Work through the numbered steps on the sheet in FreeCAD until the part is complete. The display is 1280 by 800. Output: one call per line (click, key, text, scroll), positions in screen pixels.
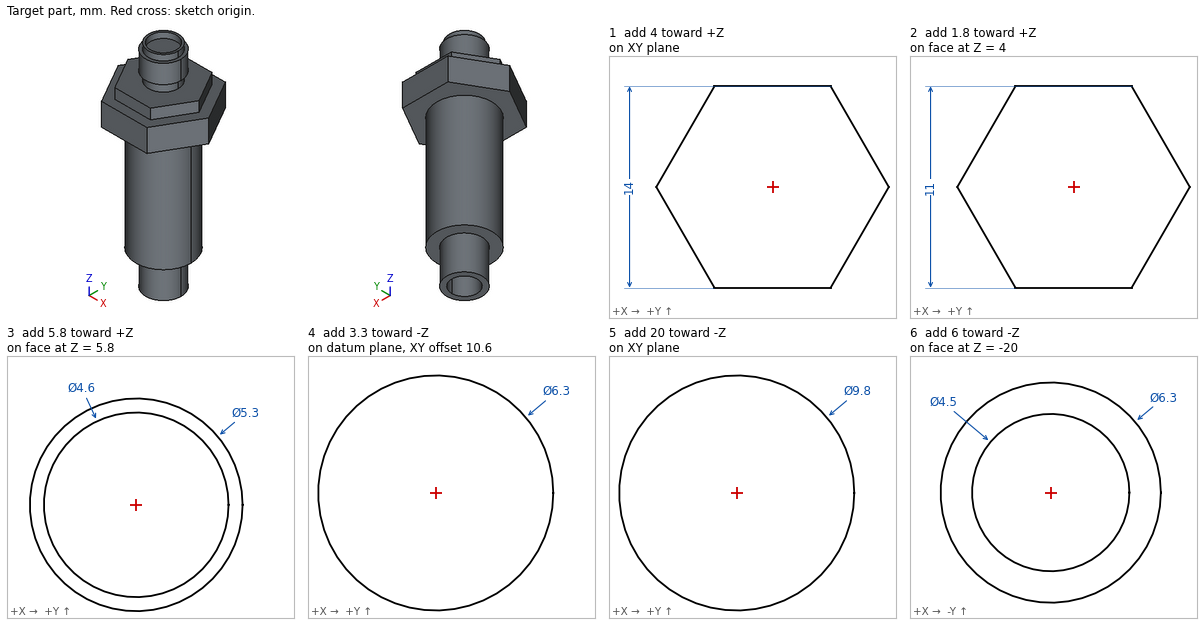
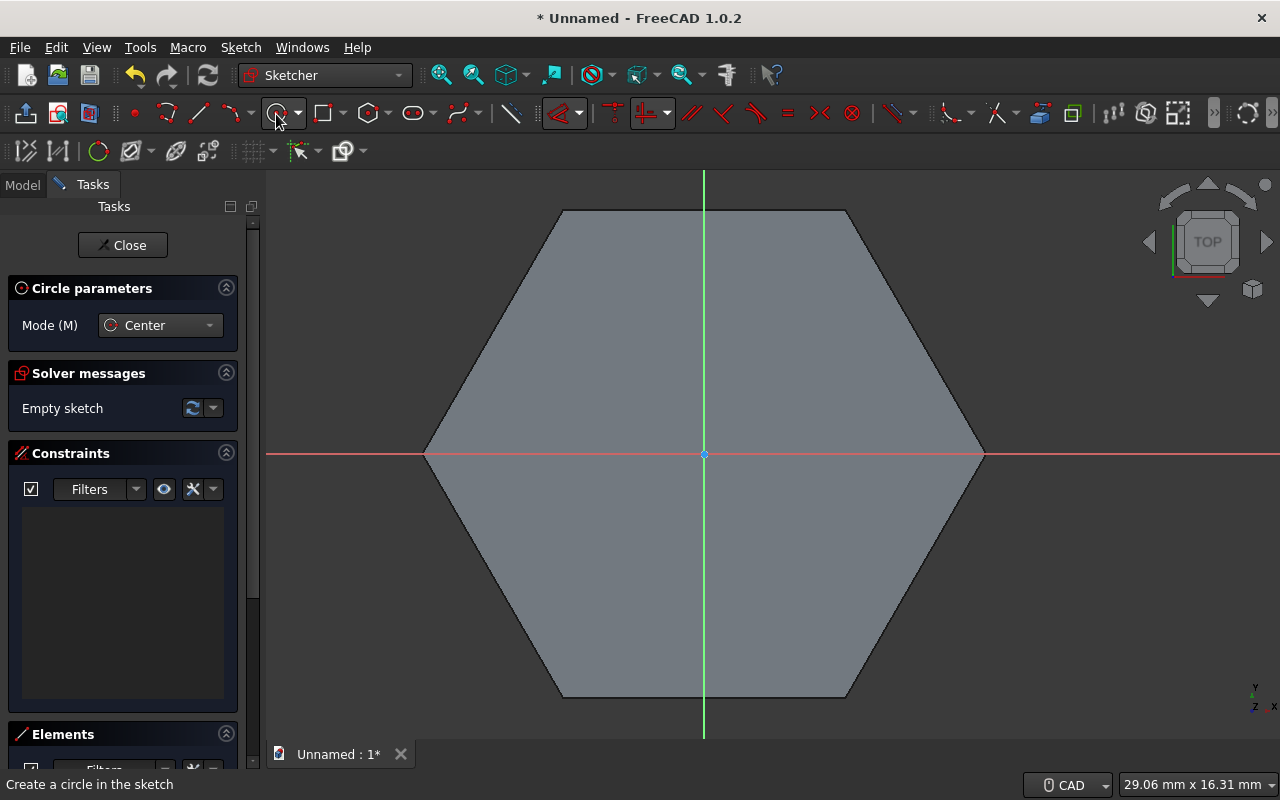
click(704, 454)
click(825, 333)
key(Escape)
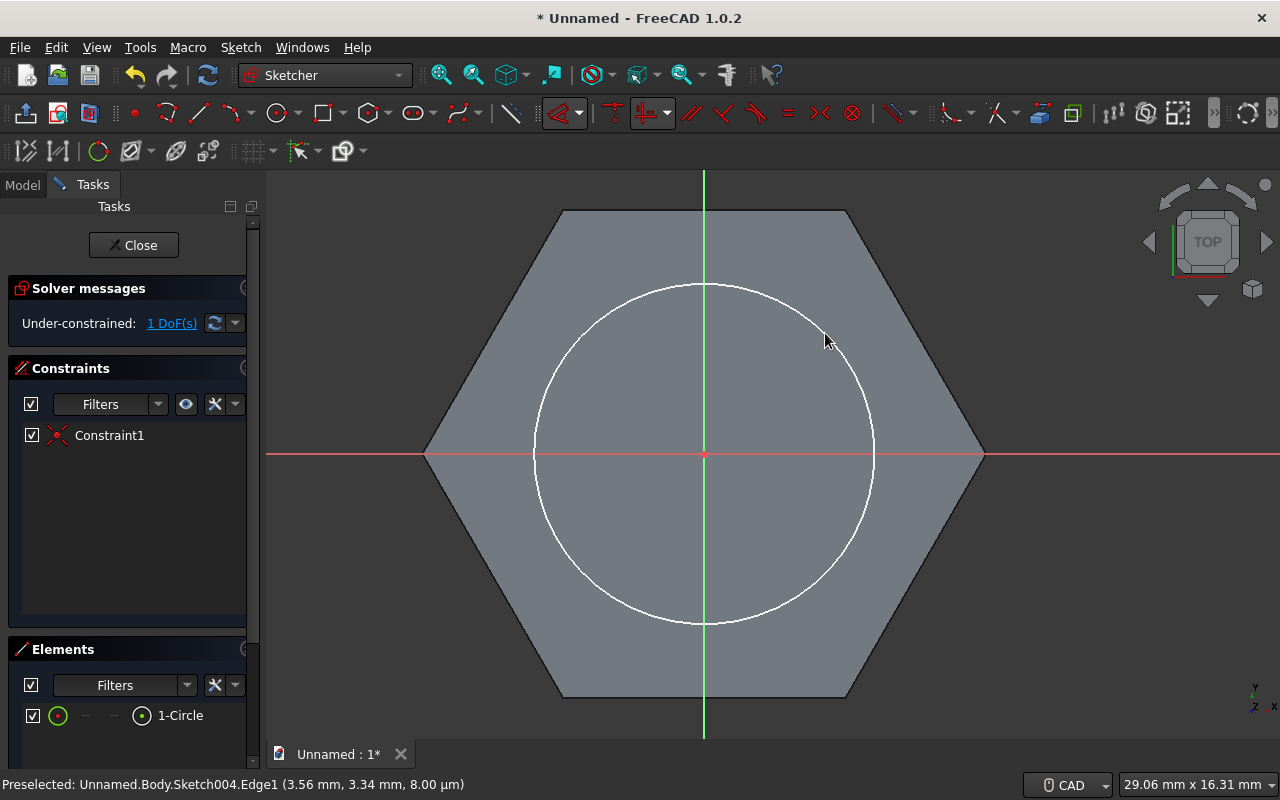
click(824, 333)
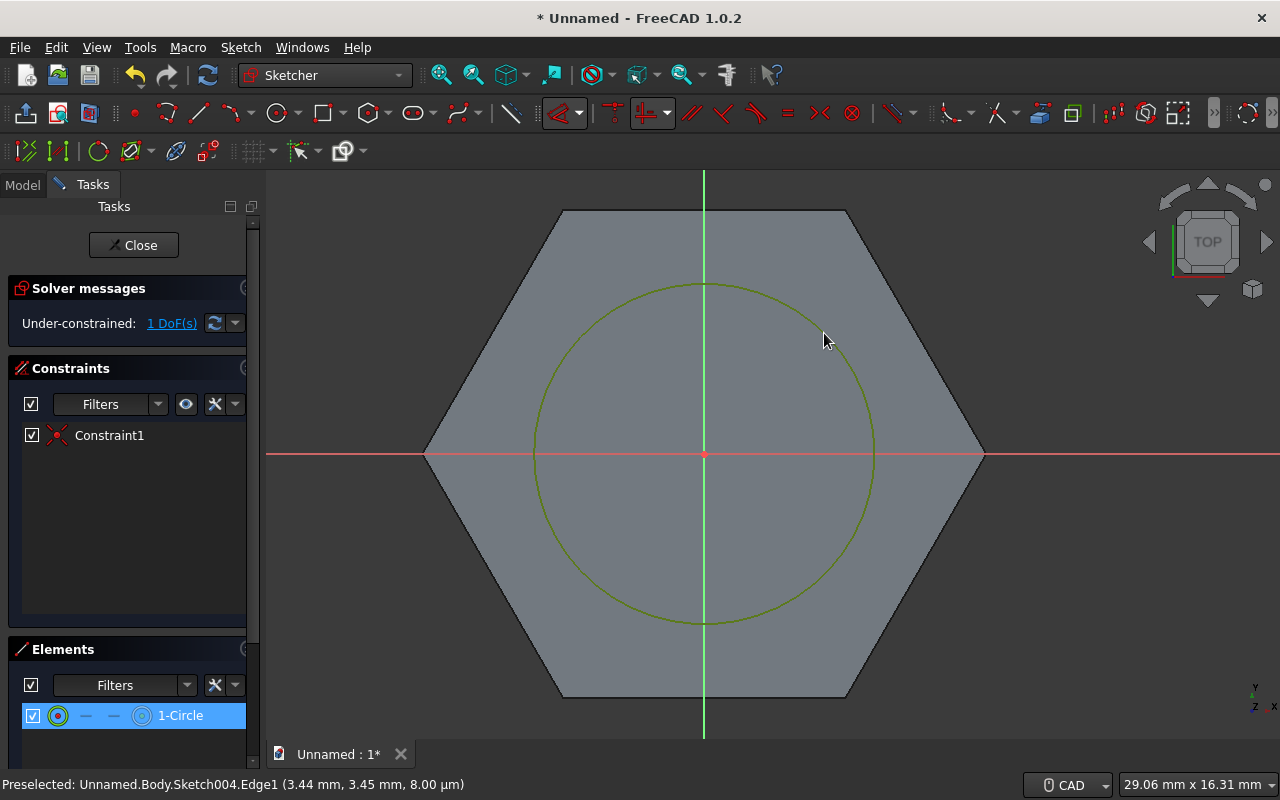
click(582, 114)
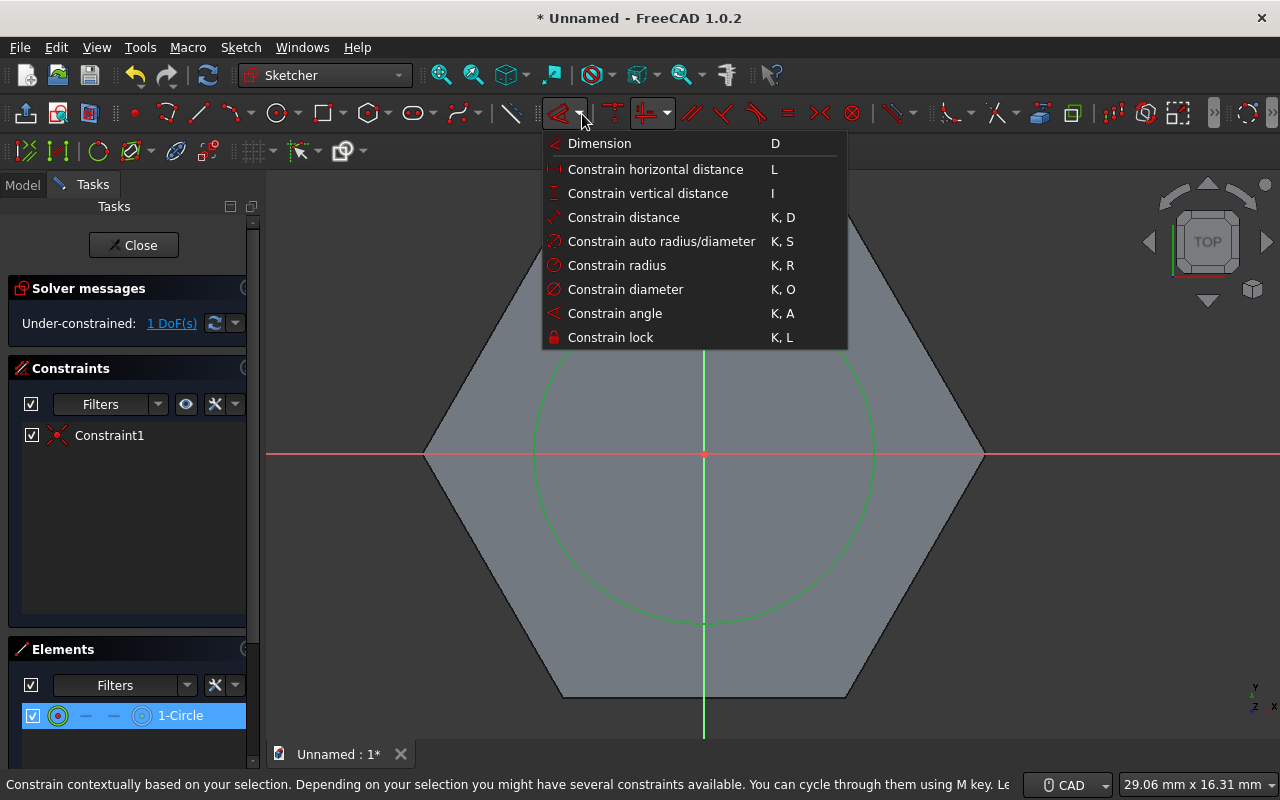
click(695, 289)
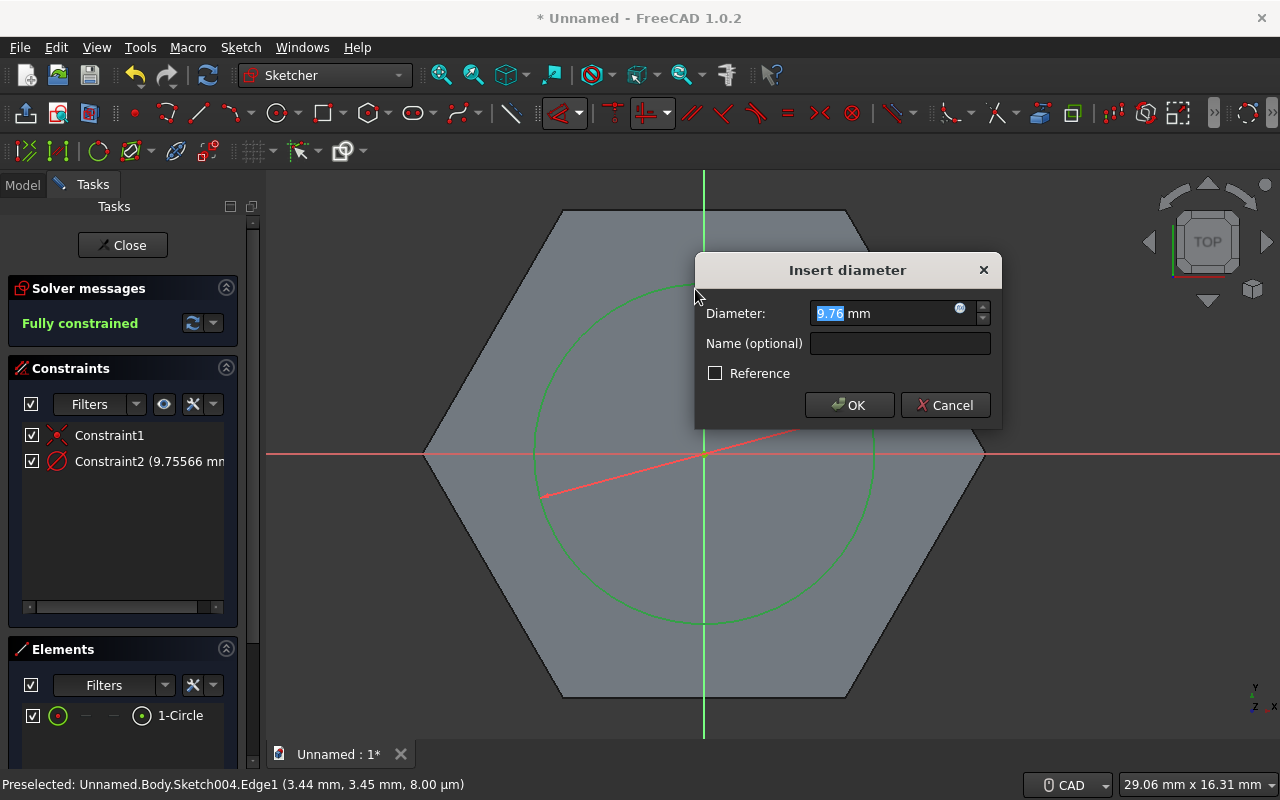
text(9.8)
key(Return)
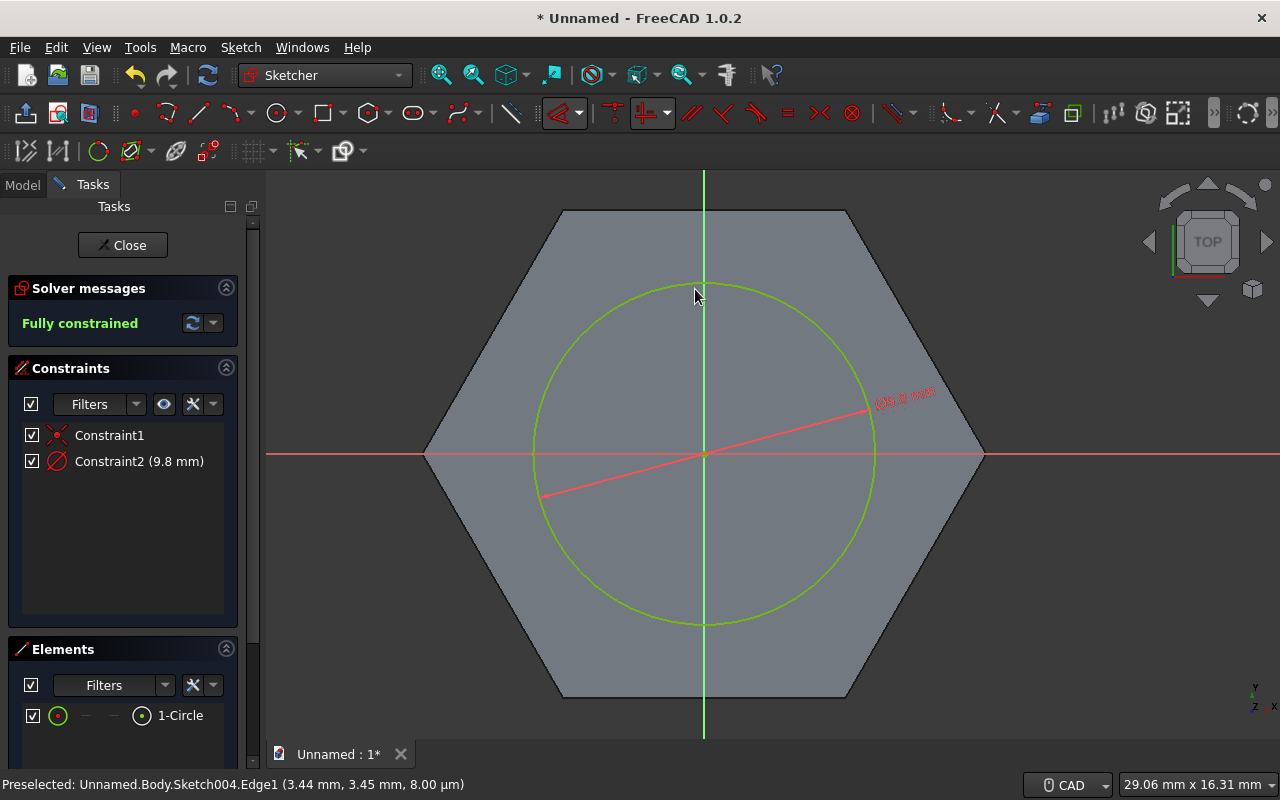
click(123, 245)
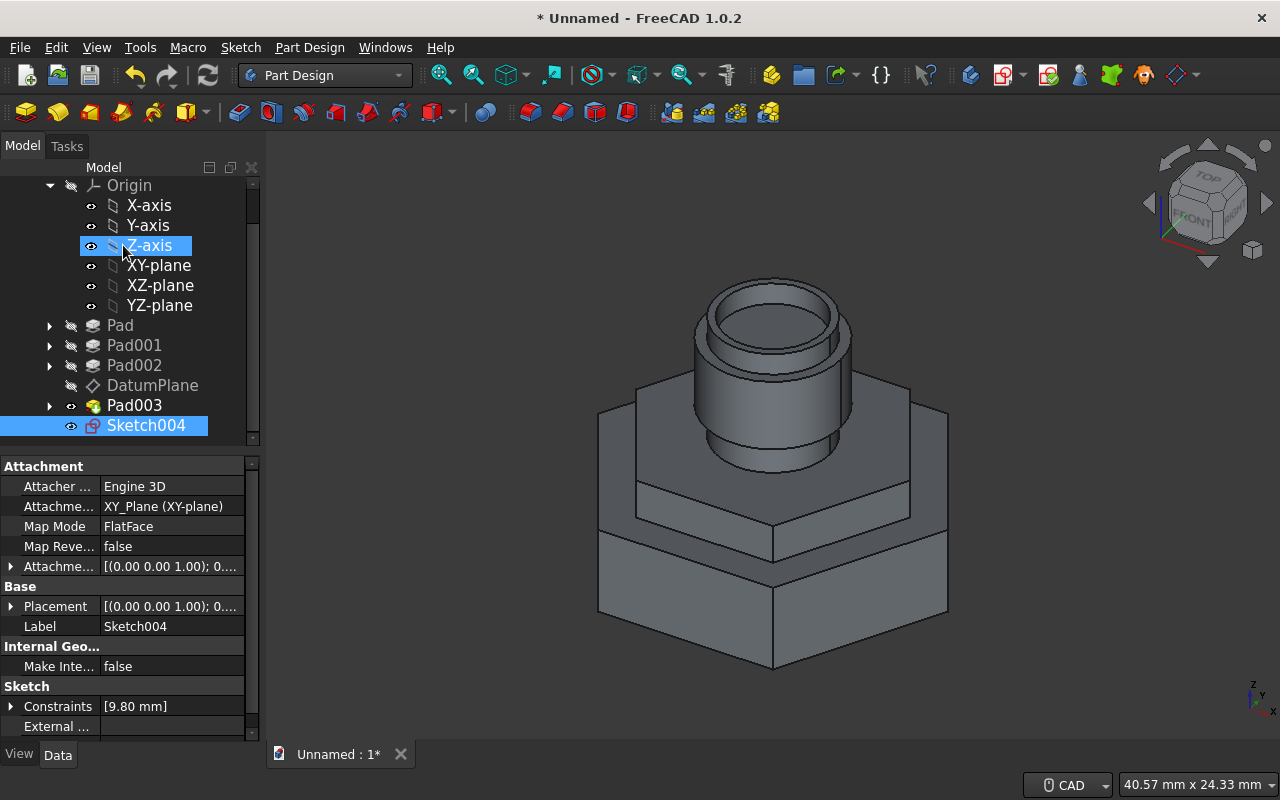
click(26, 112)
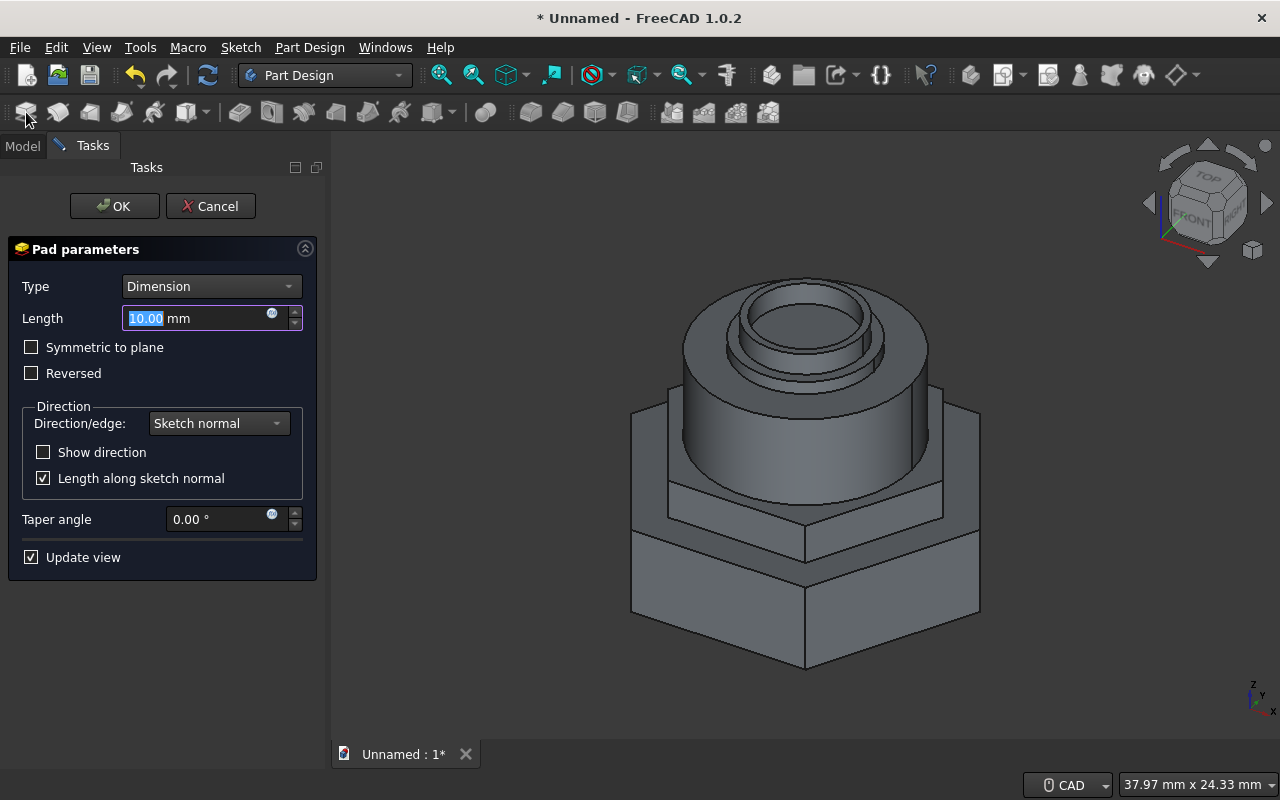
text(20)
key(Tab)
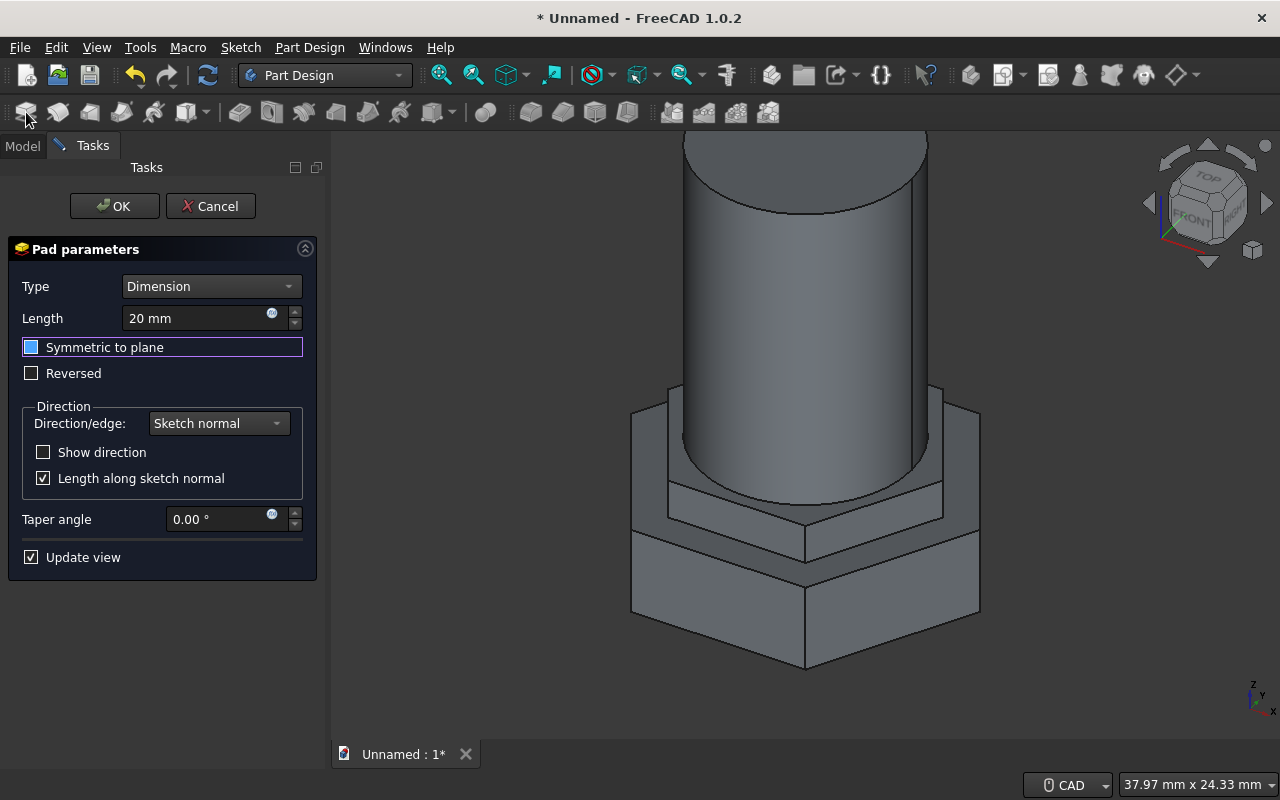
click(30, 373)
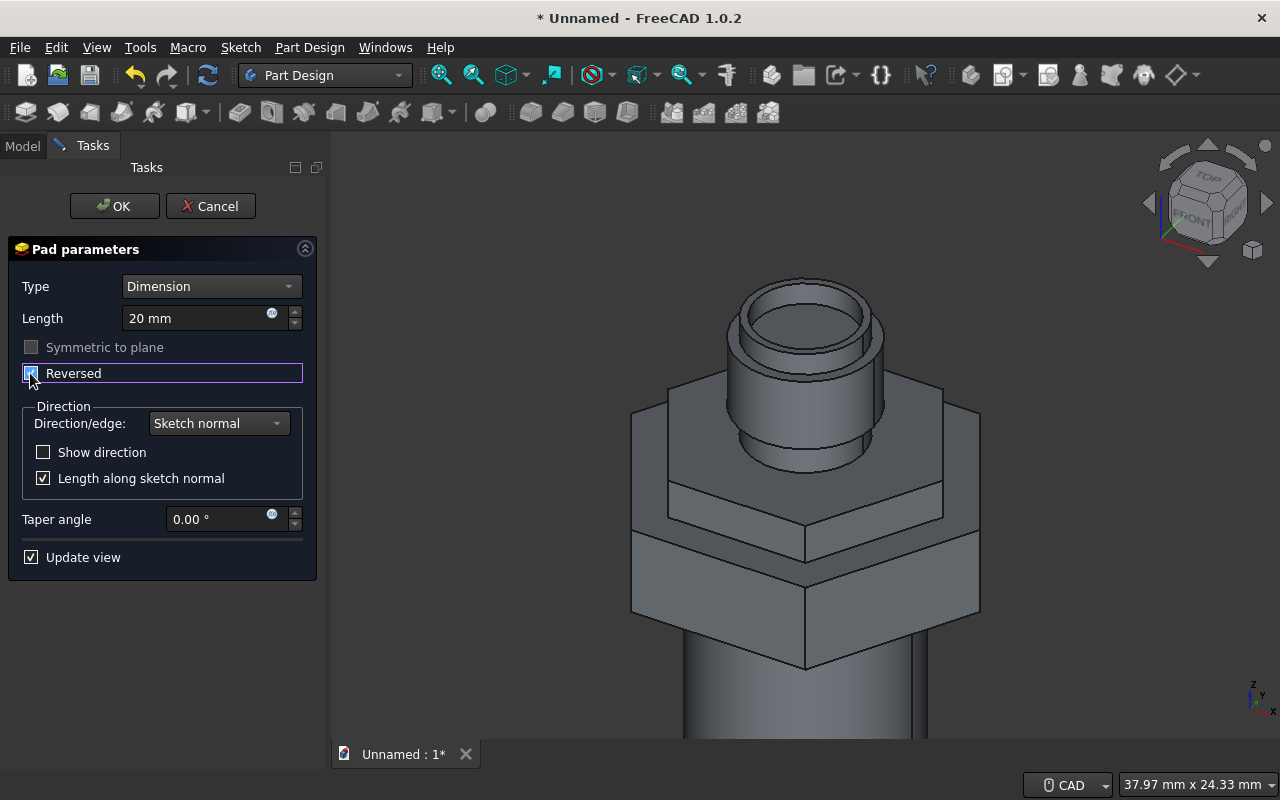
click(115, 206)